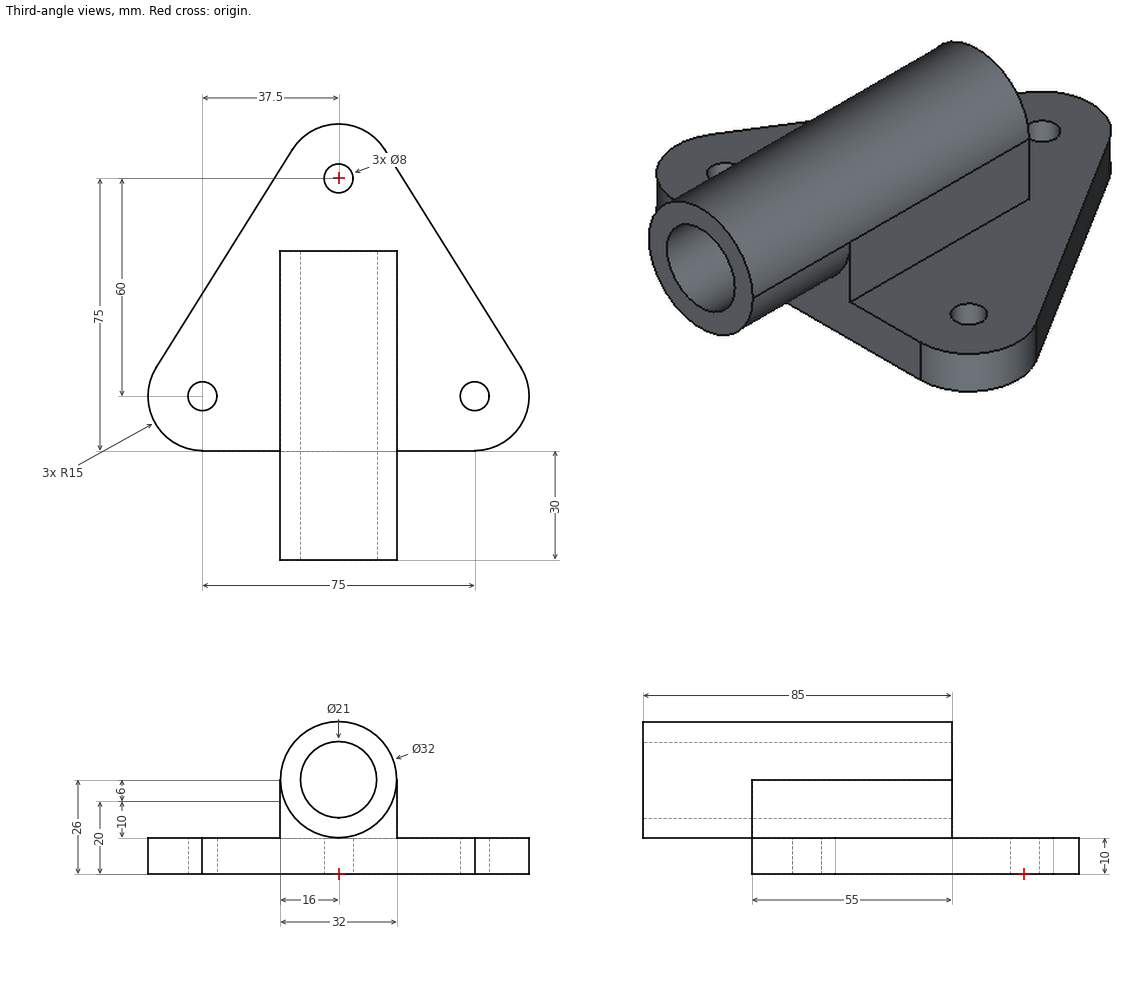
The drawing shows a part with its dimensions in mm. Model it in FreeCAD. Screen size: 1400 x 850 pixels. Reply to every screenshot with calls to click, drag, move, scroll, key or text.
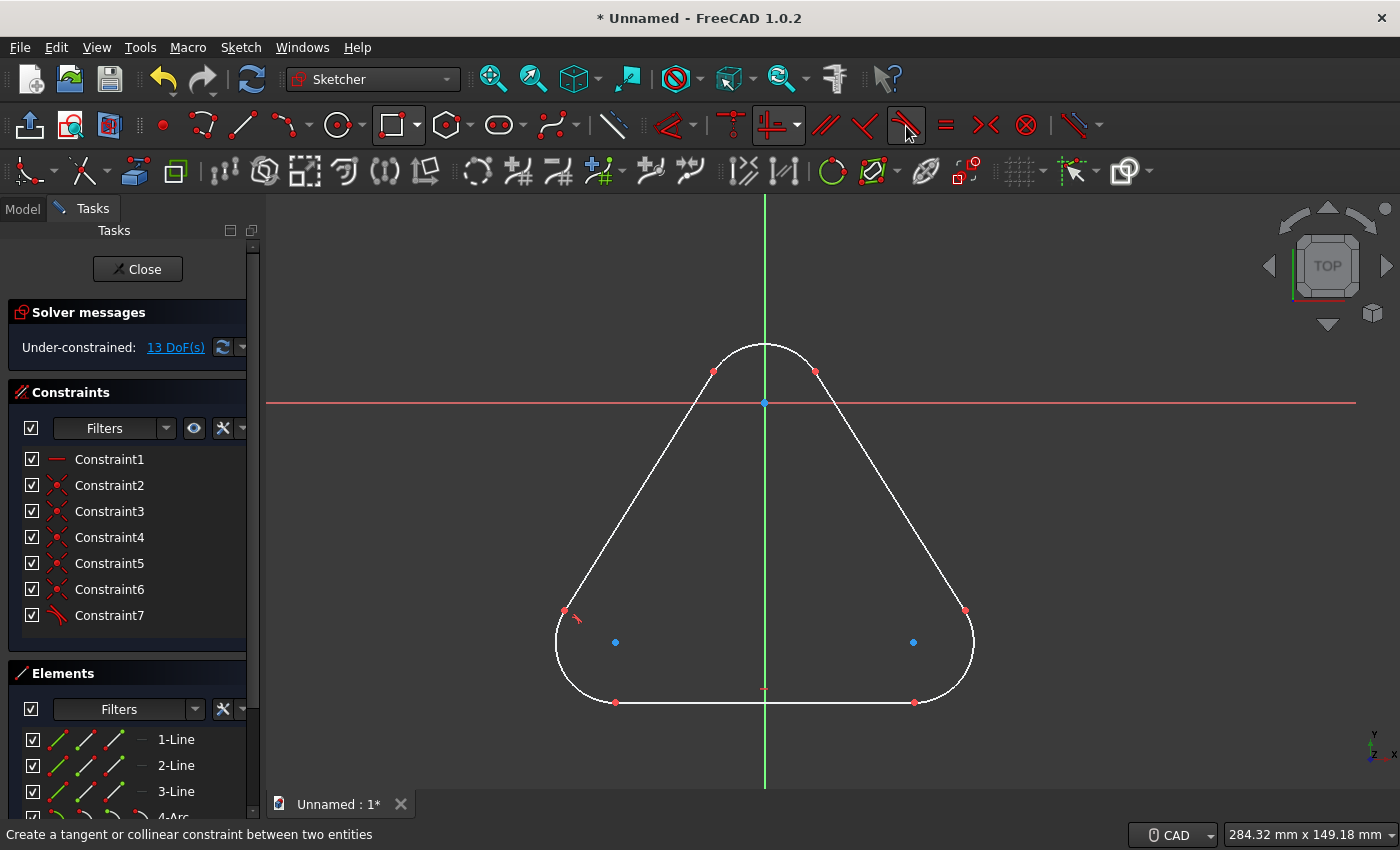
click(669, 444)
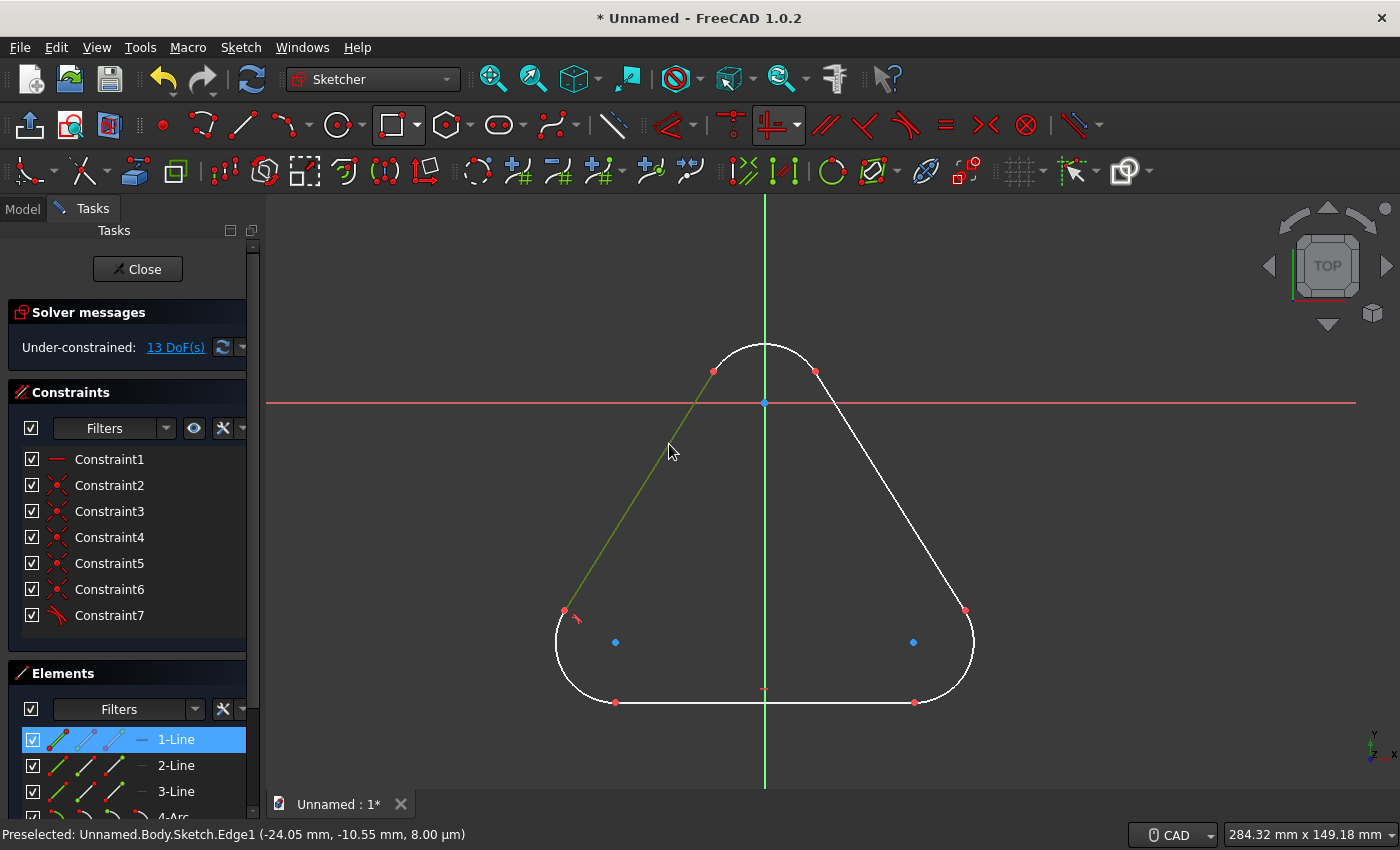
click(788, 349)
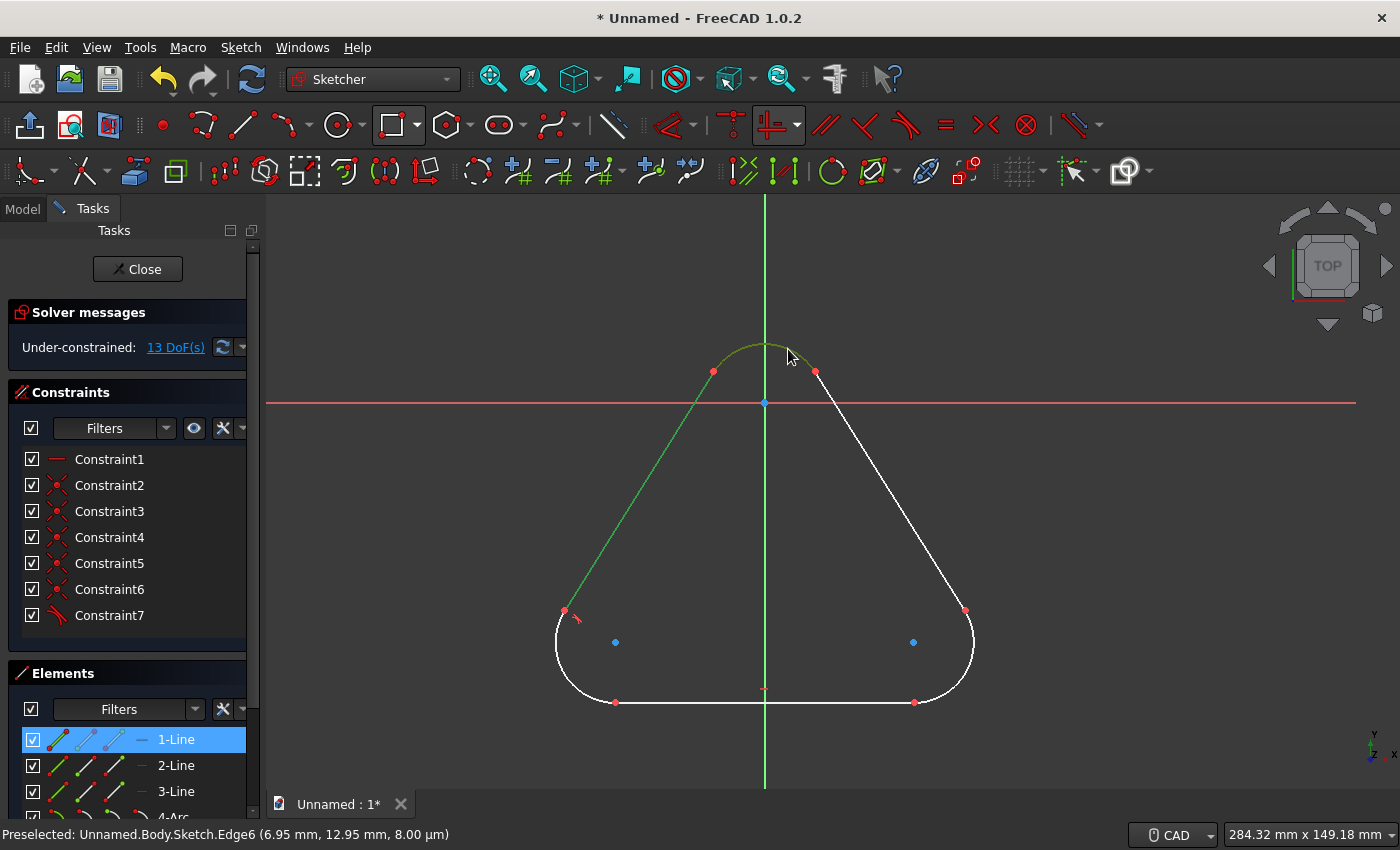
click(906, 126)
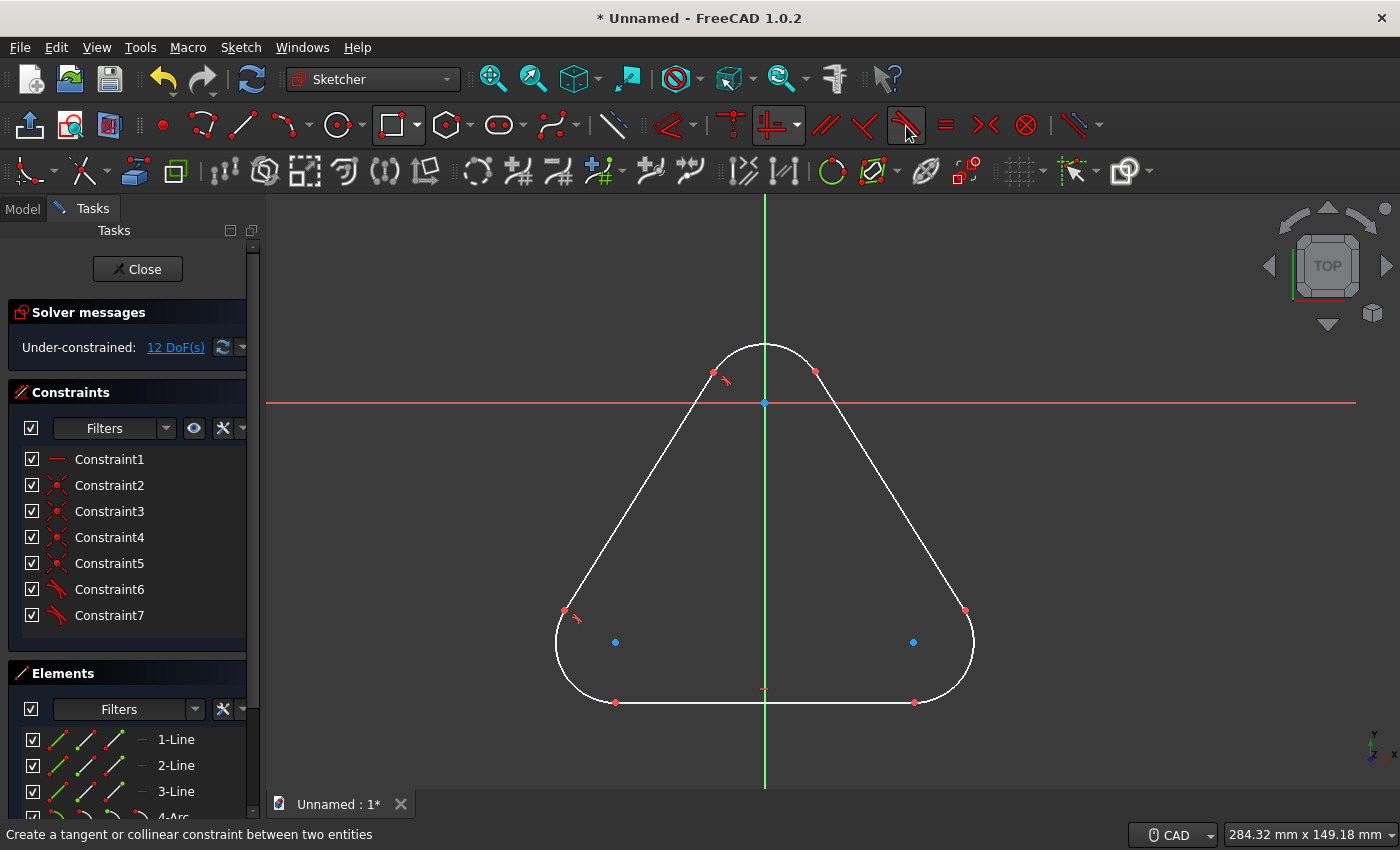
click(705, 703)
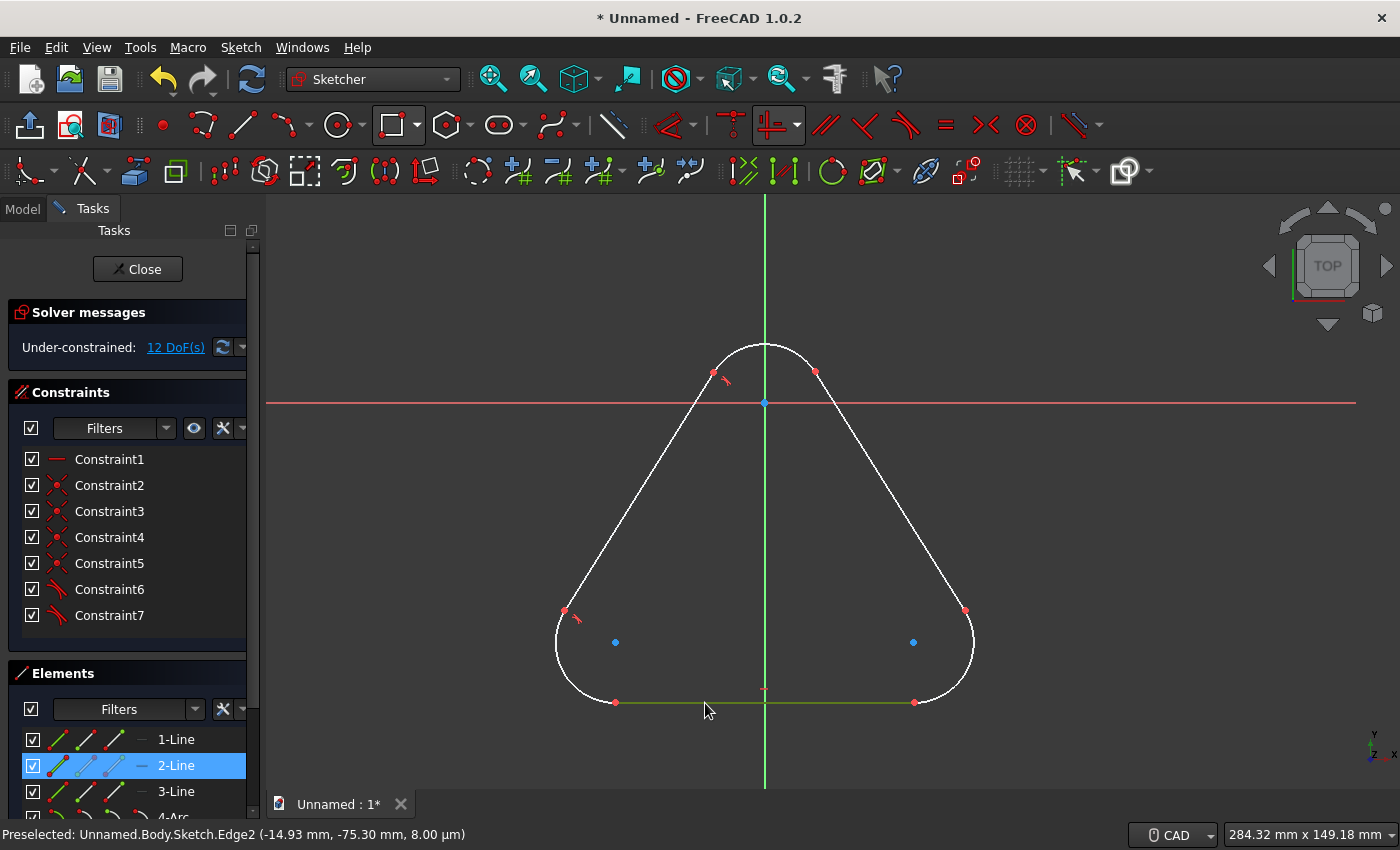
click(556, 647)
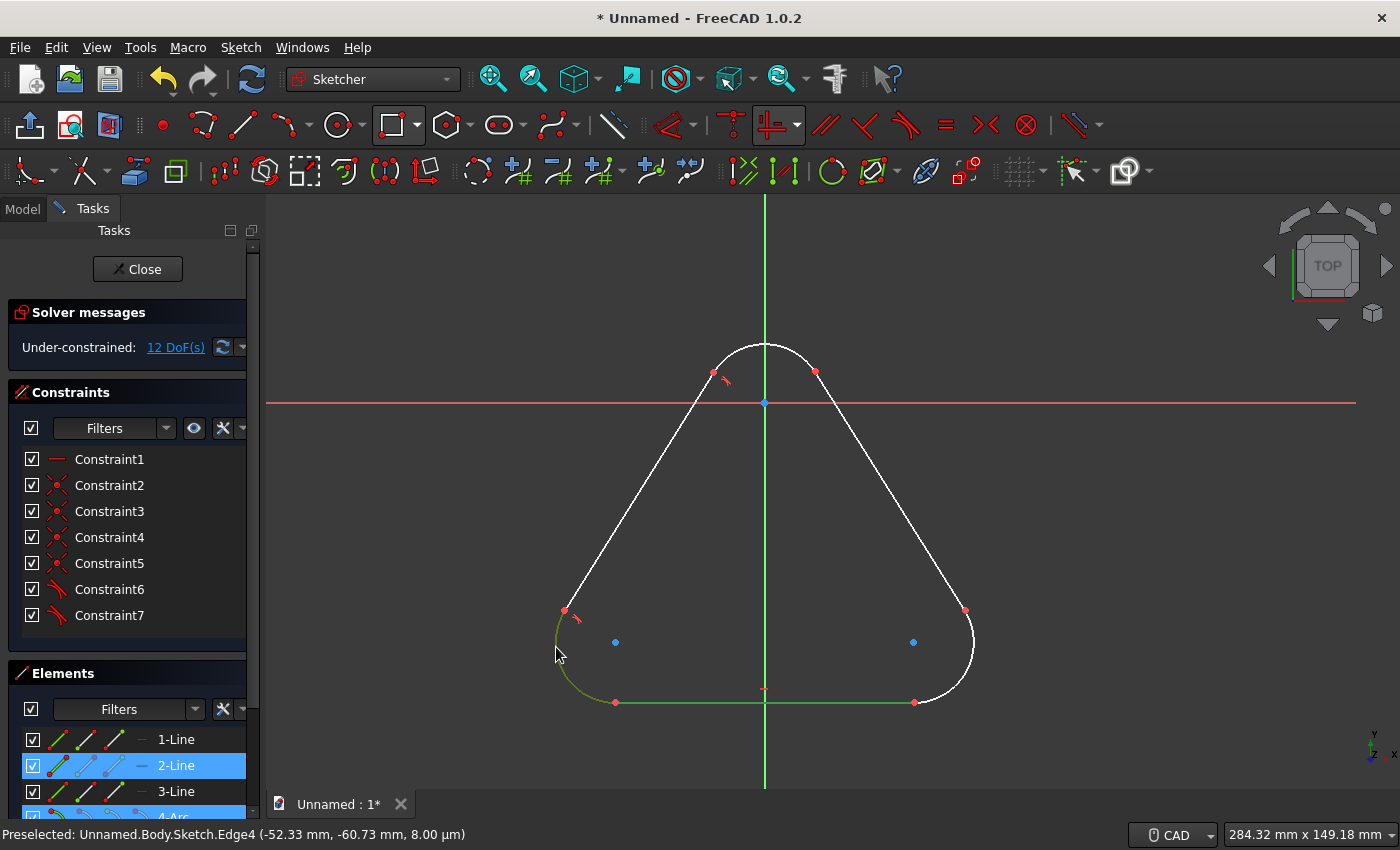
click(906, 126)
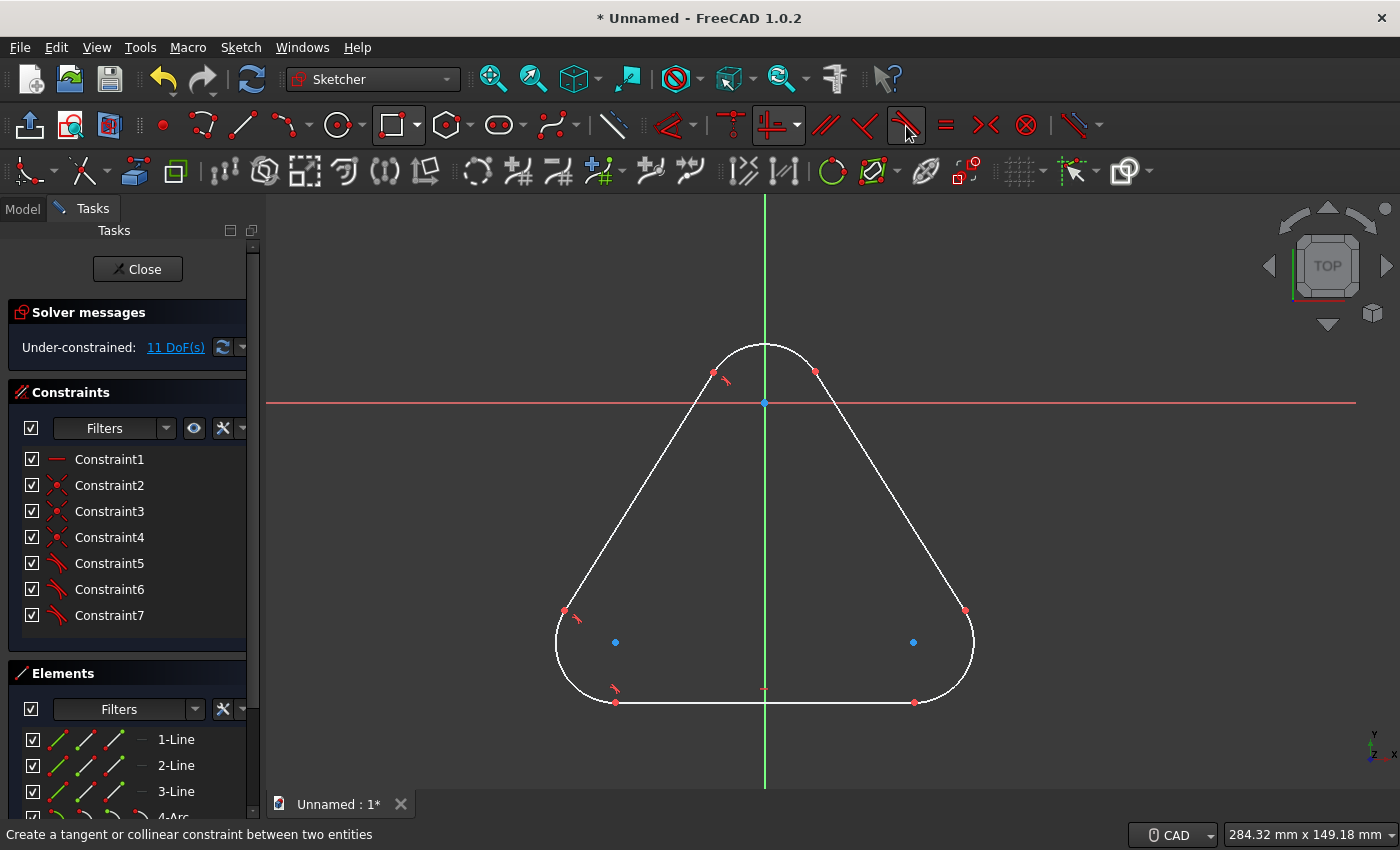
click(705, 703)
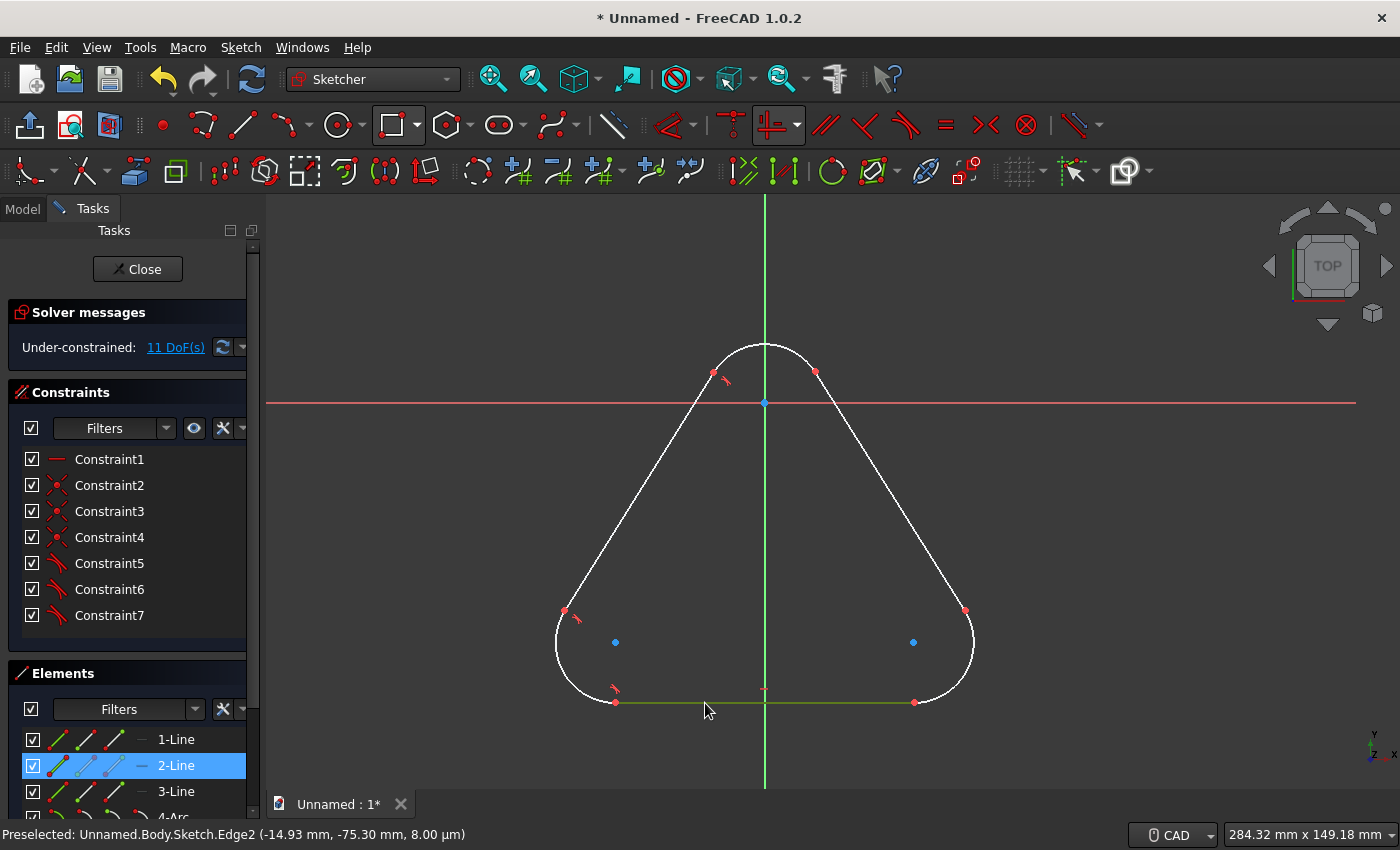
click(950, 691)